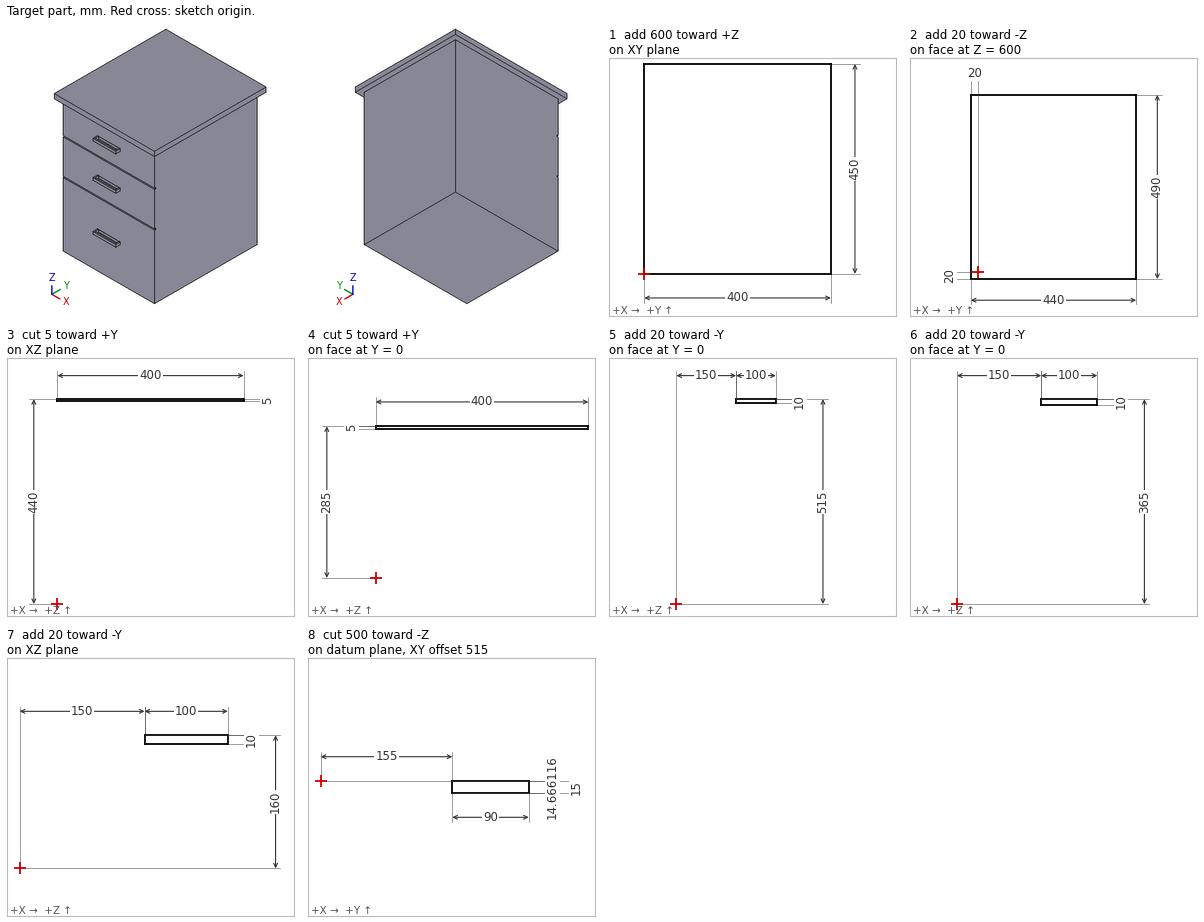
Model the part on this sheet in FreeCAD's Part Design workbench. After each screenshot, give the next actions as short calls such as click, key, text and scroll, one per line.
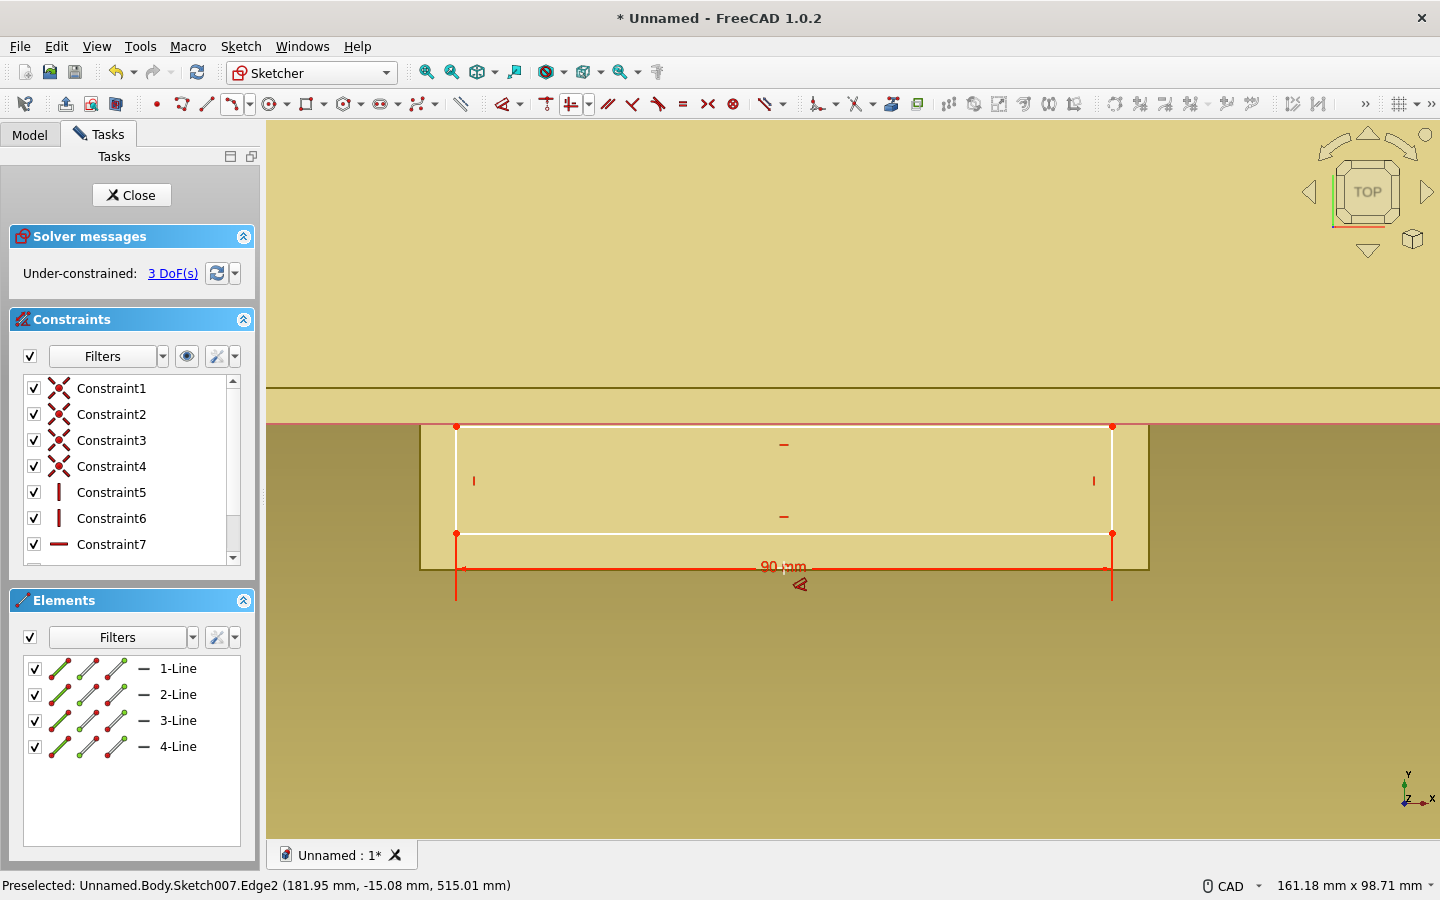
click(456, 534)
click(490, 479)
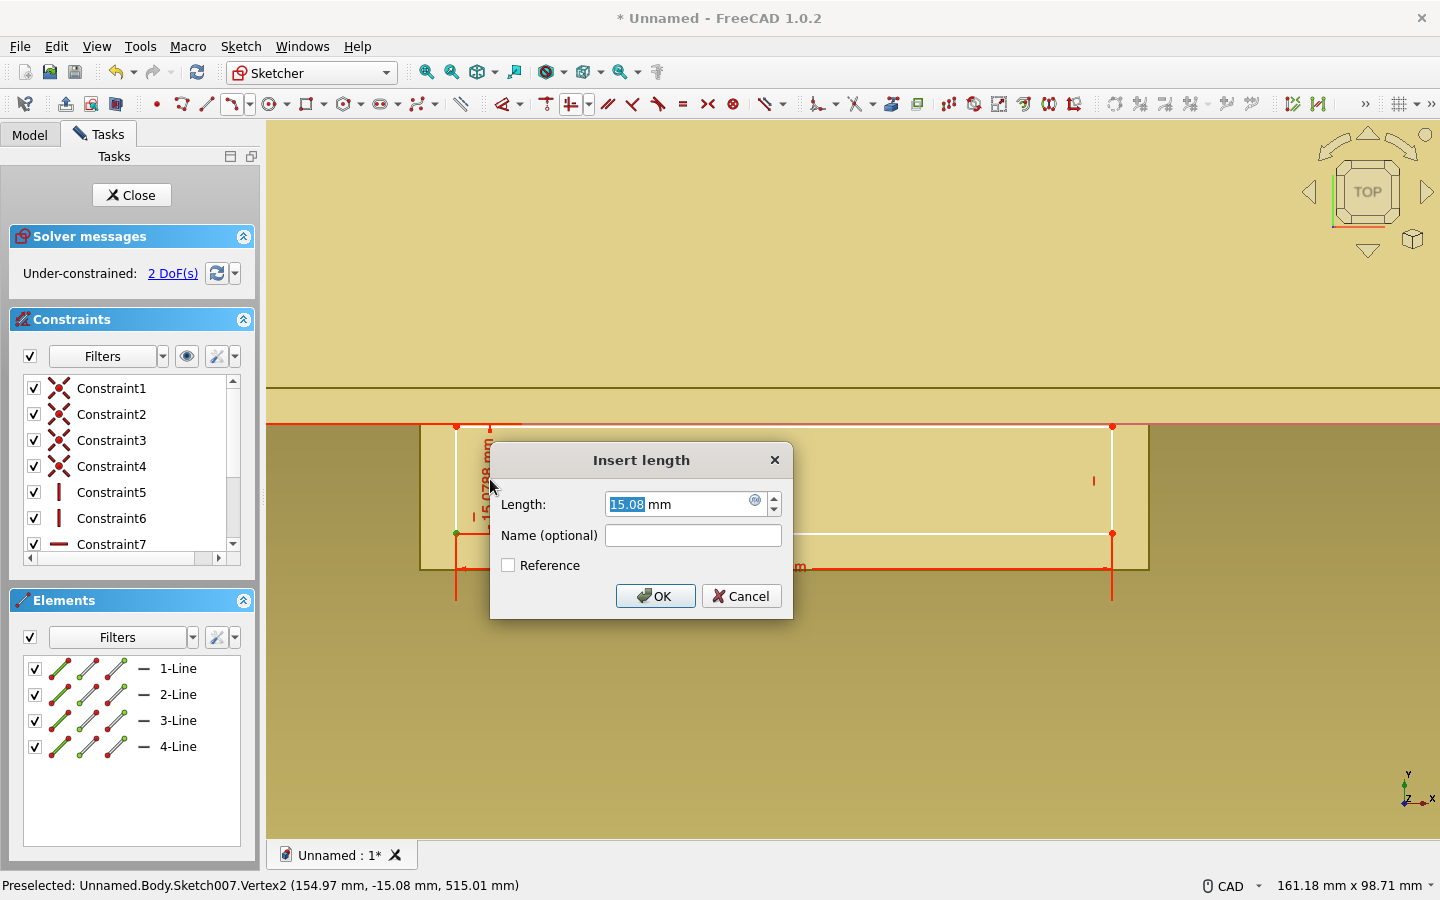
text(15)
key(Return)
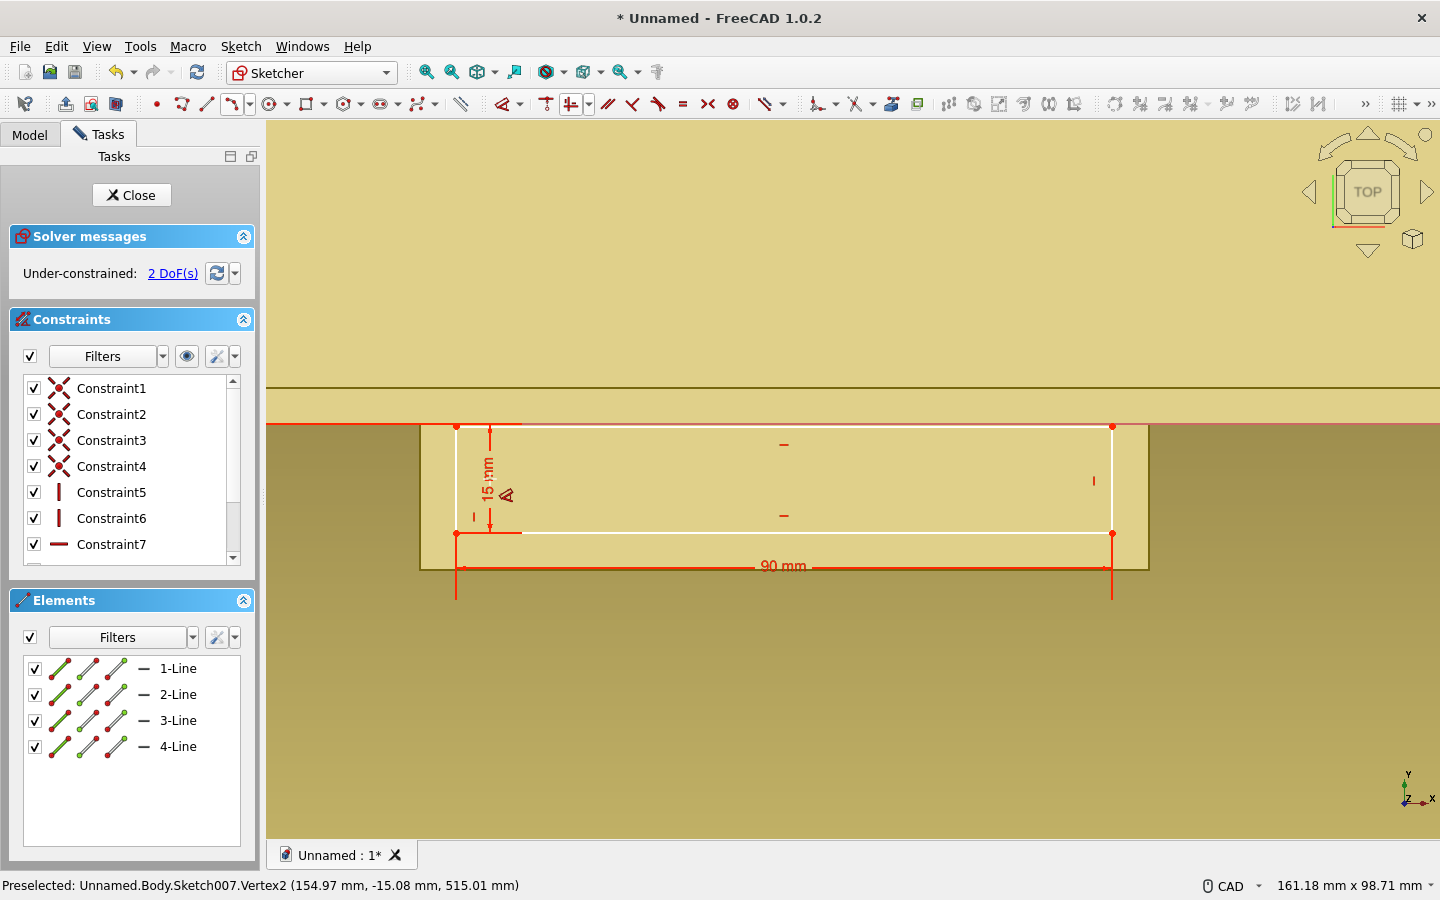
click(456, 427)
click(375, 390)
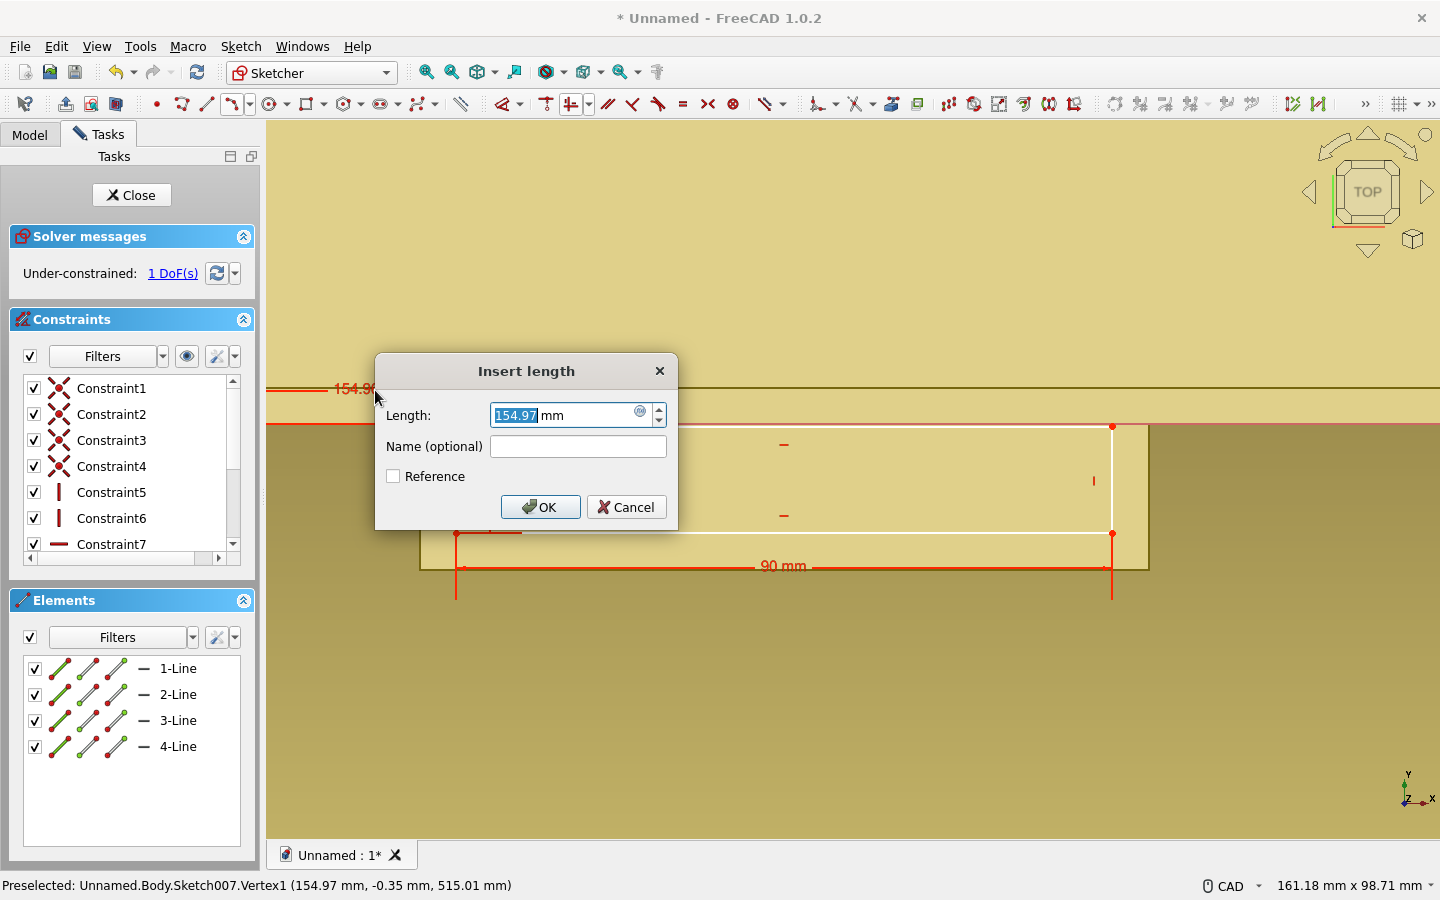
text(155)
key(Return)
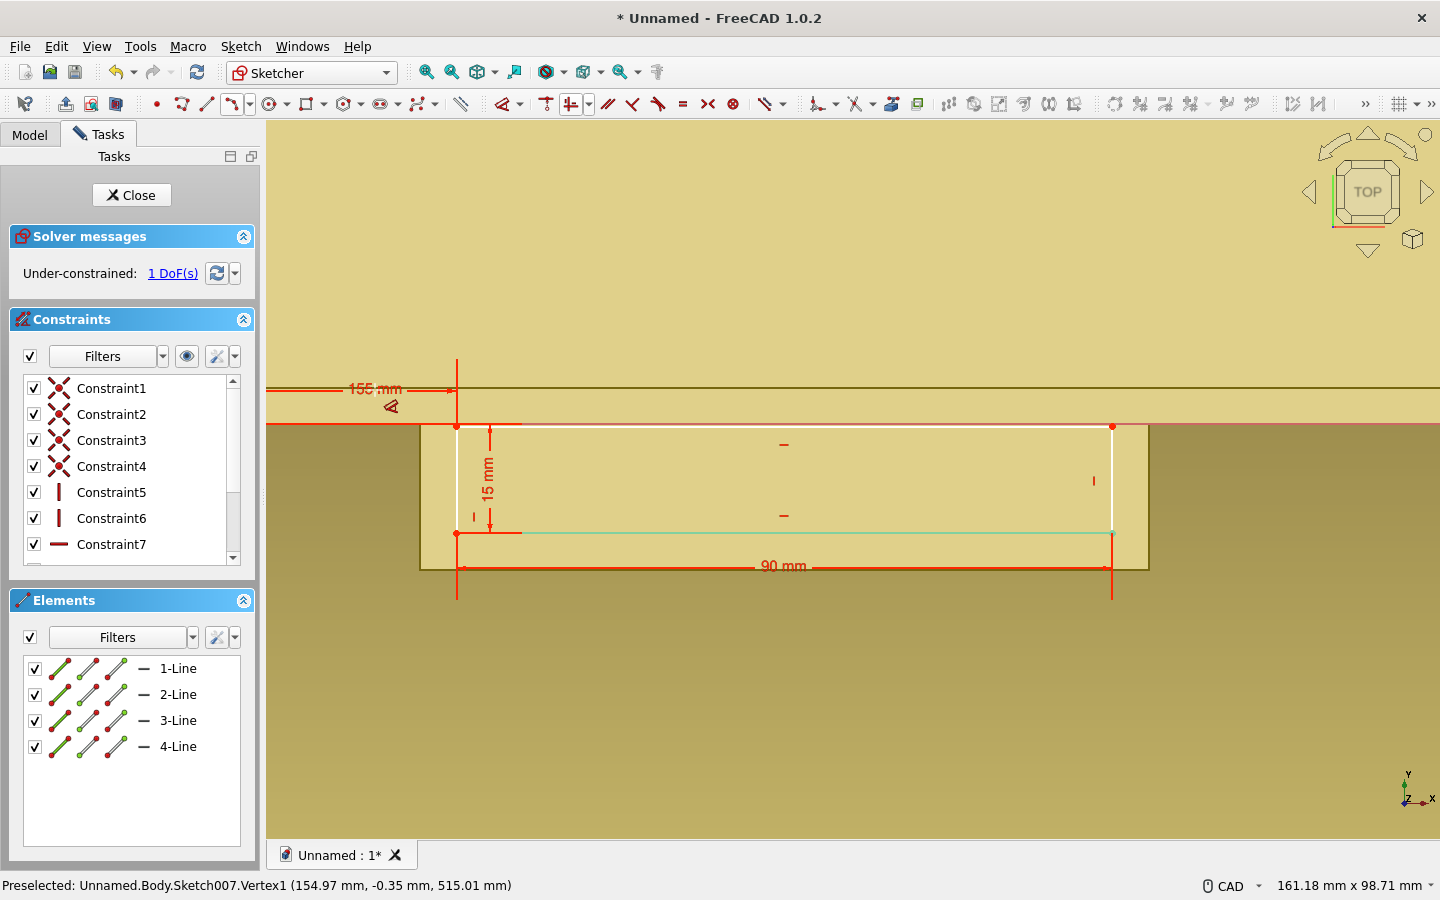
click(457, 459)
click(423, 456)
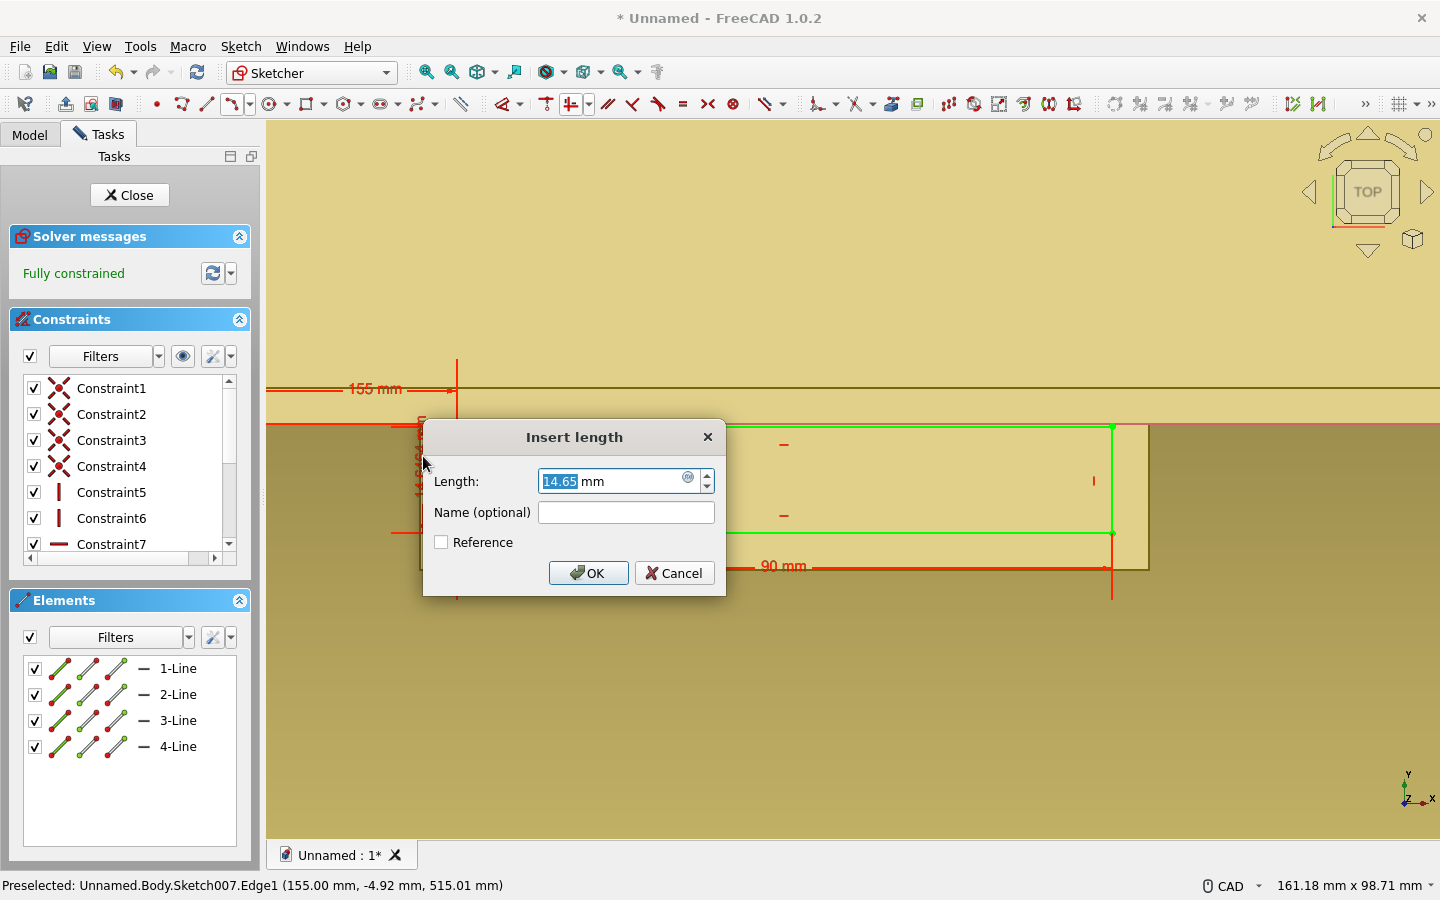
text(14.666116)
key(Return)
key(Escape)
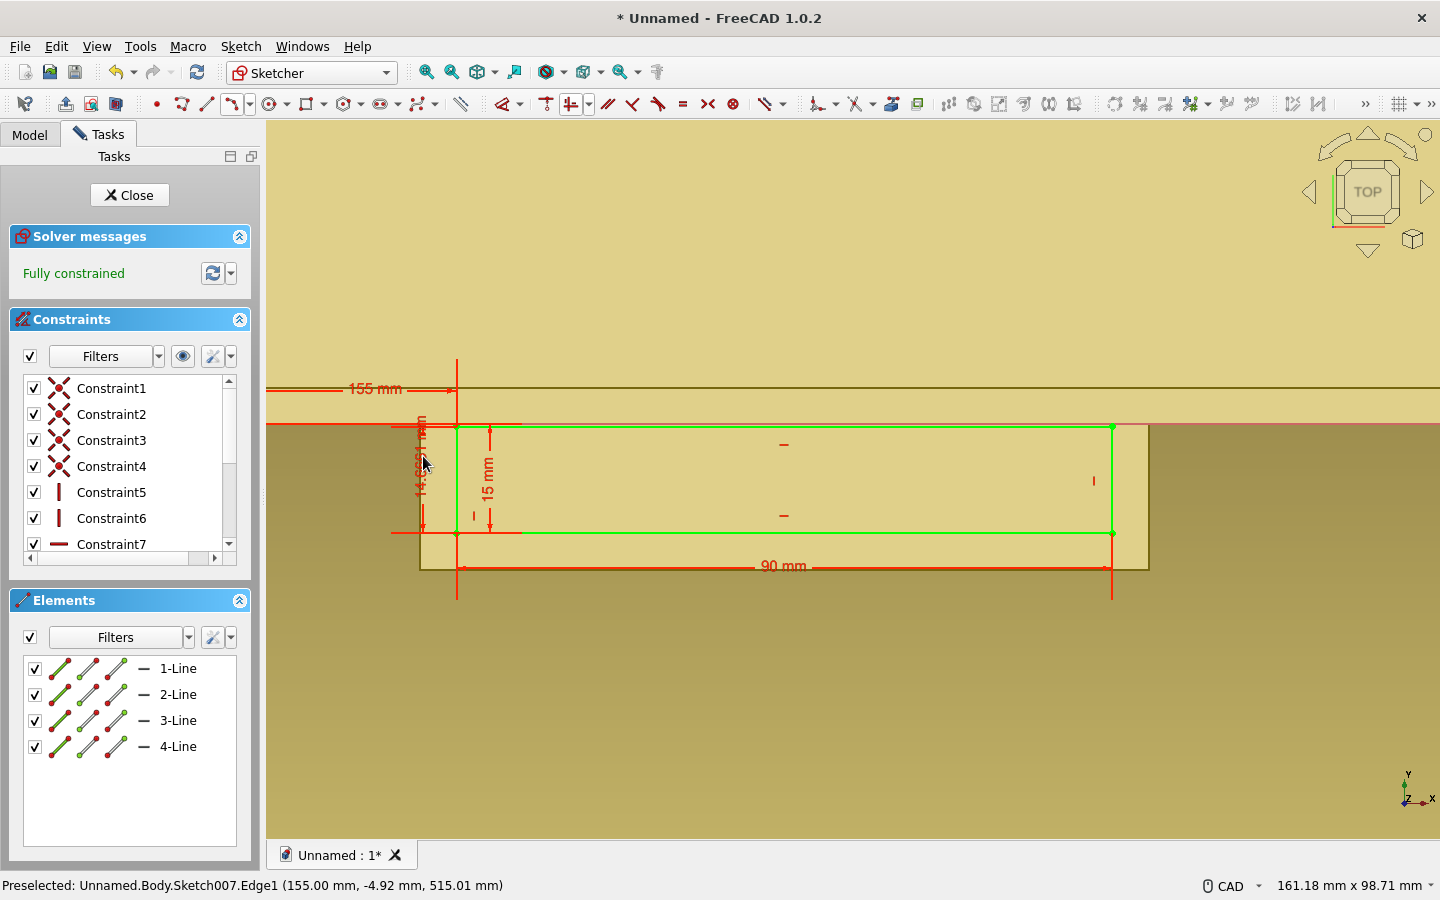
click(130, 195)